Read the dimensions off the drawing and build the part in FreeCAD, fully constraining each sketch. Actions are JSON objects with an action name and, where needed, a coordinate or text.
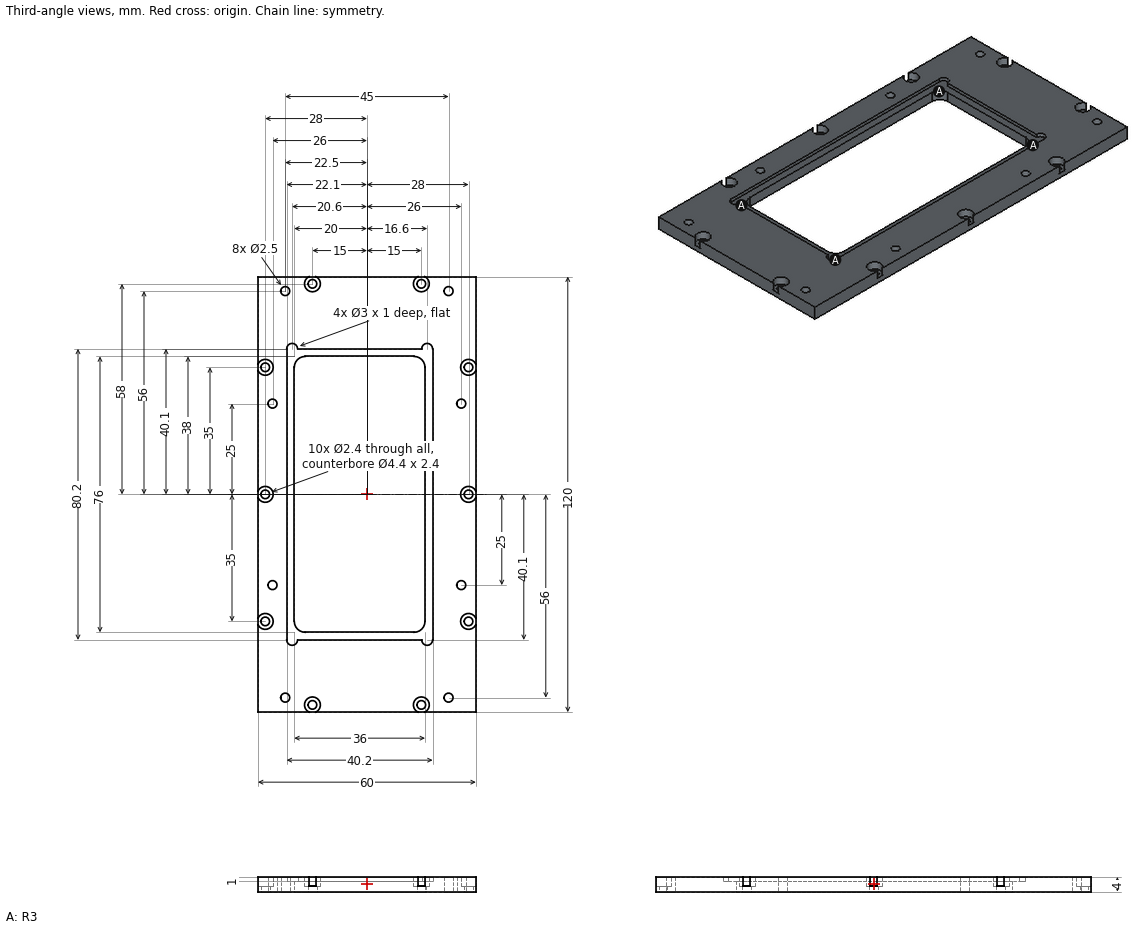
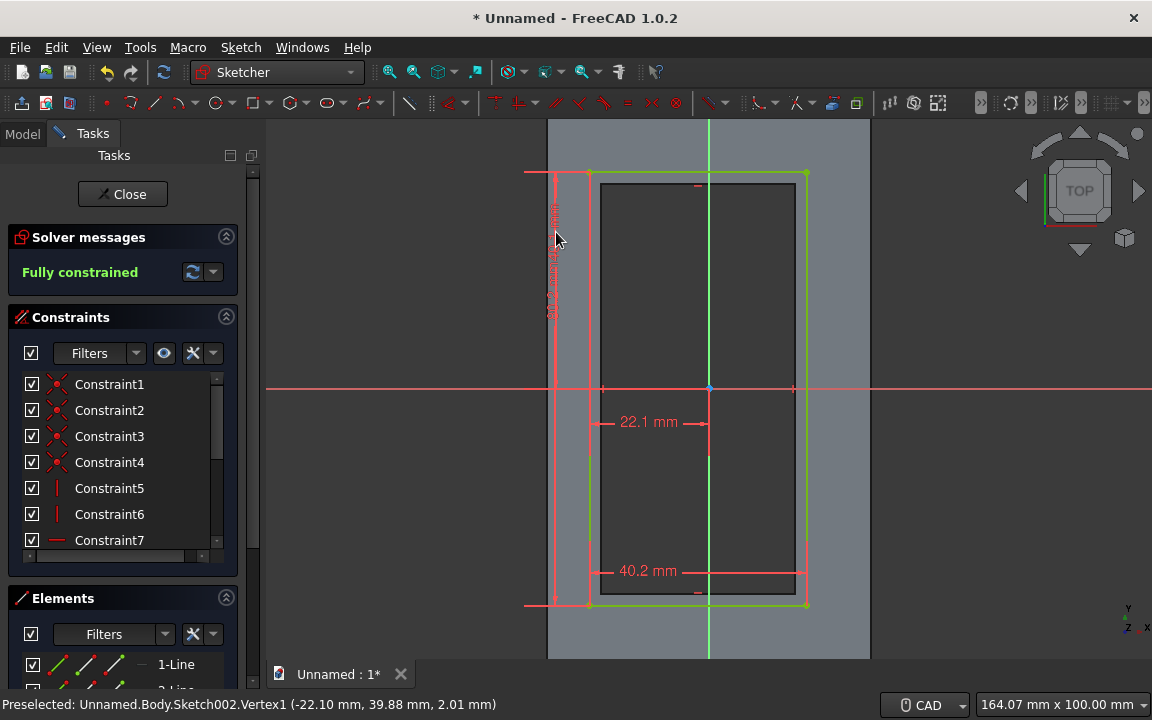
{"action": "left_click", "coordinate": [123, 194]}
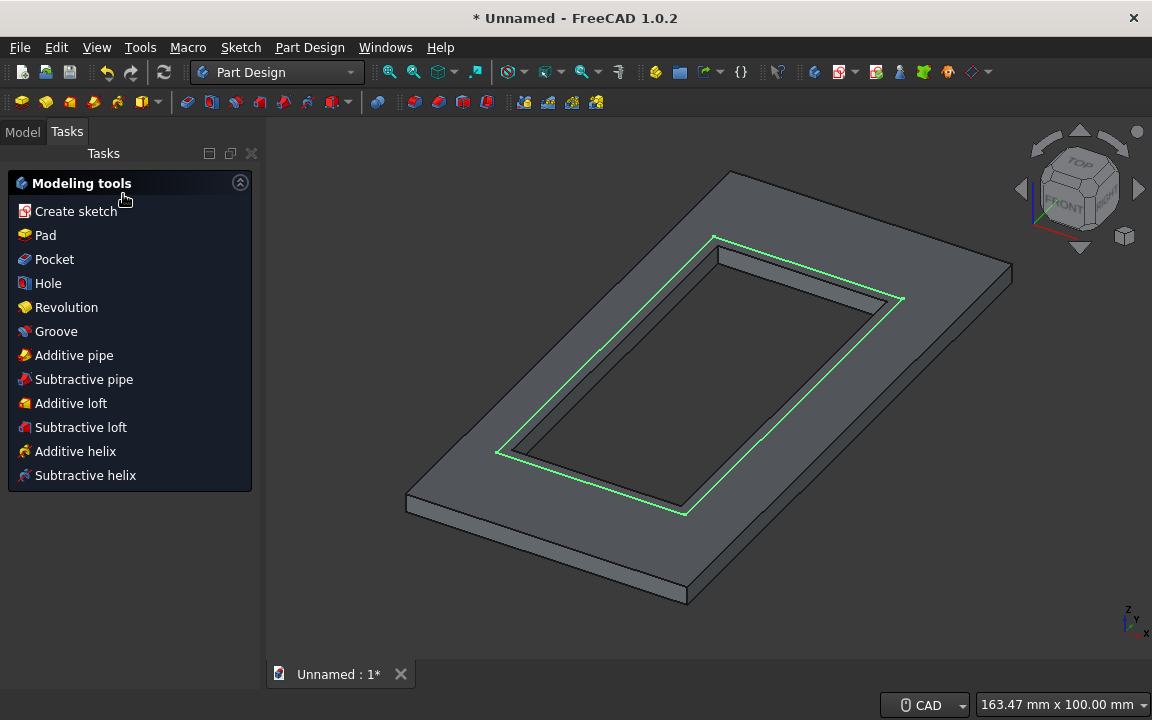
{"action": "left_click", "coordinate": [188, 102]}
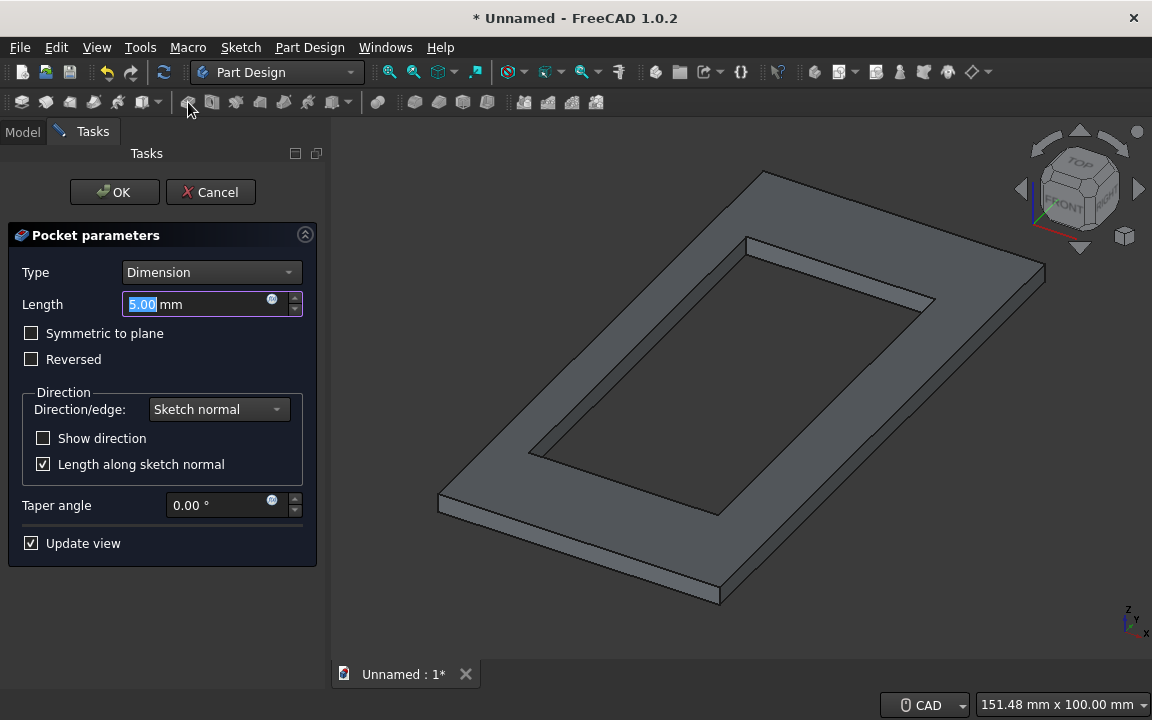
{"action": "type", "text": "1"}
{"action": "key", "text": "Tab"}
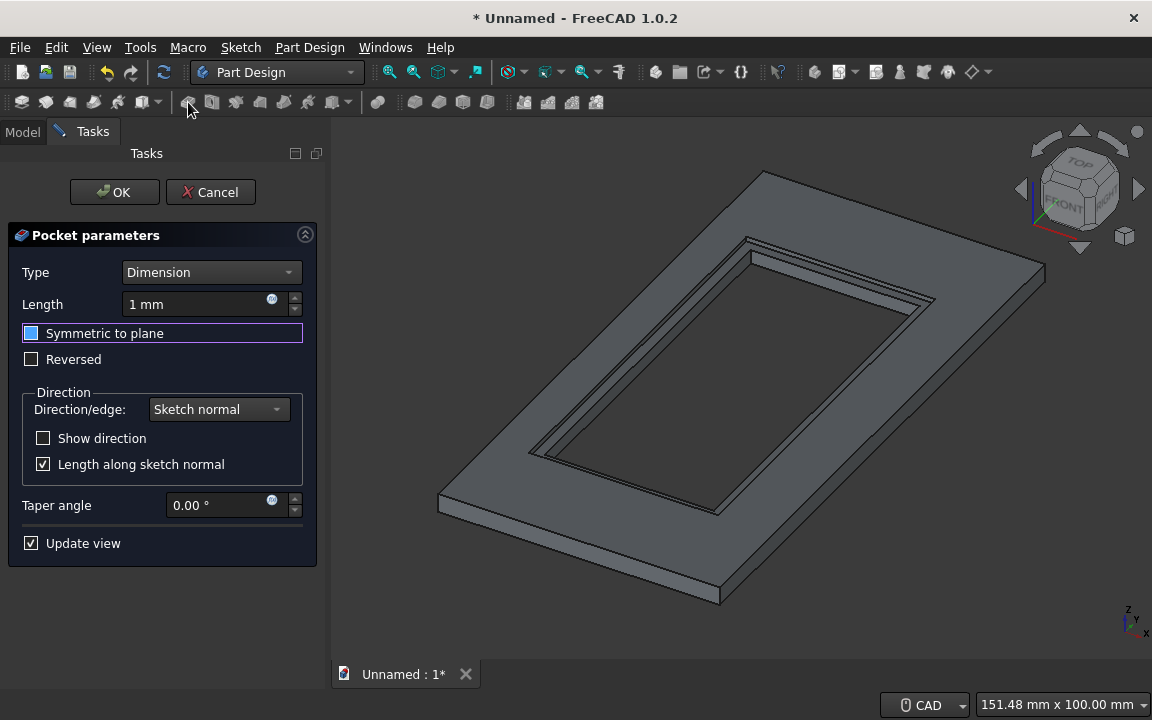
{"action": "left_click", "coordinate": [115, 192]}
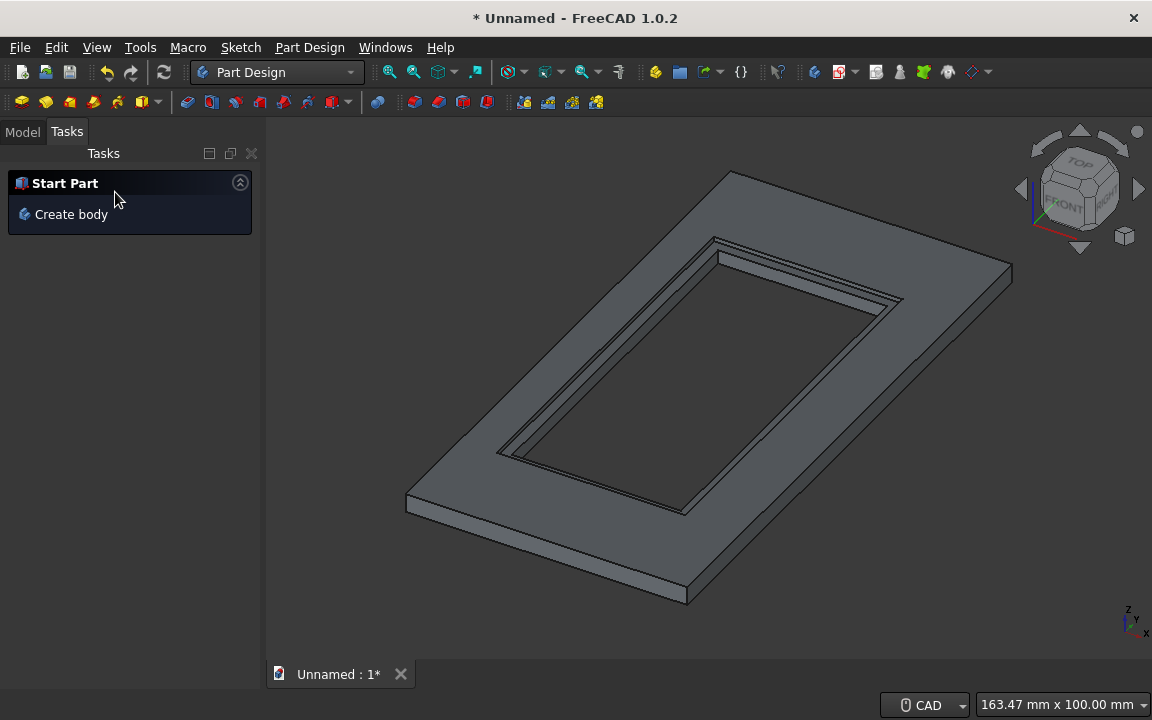
{"action": "left_click", "coordinate": [929, 266]}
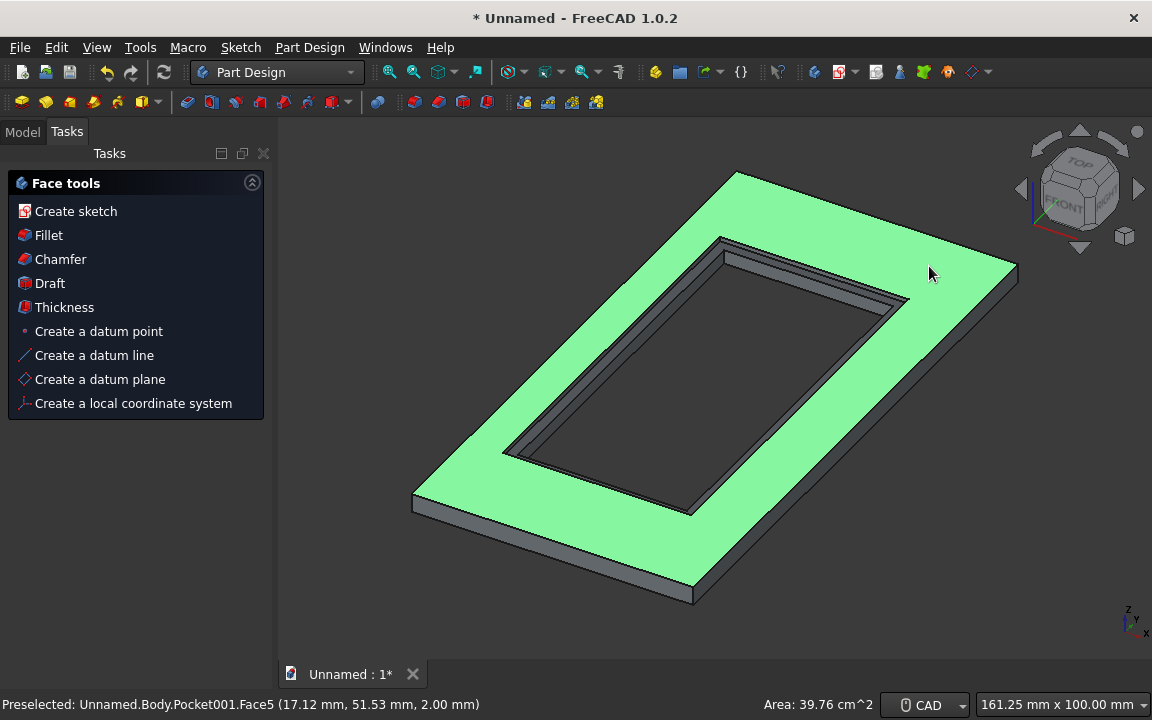
{"action": "left_click", "coordinate": [840, 72]}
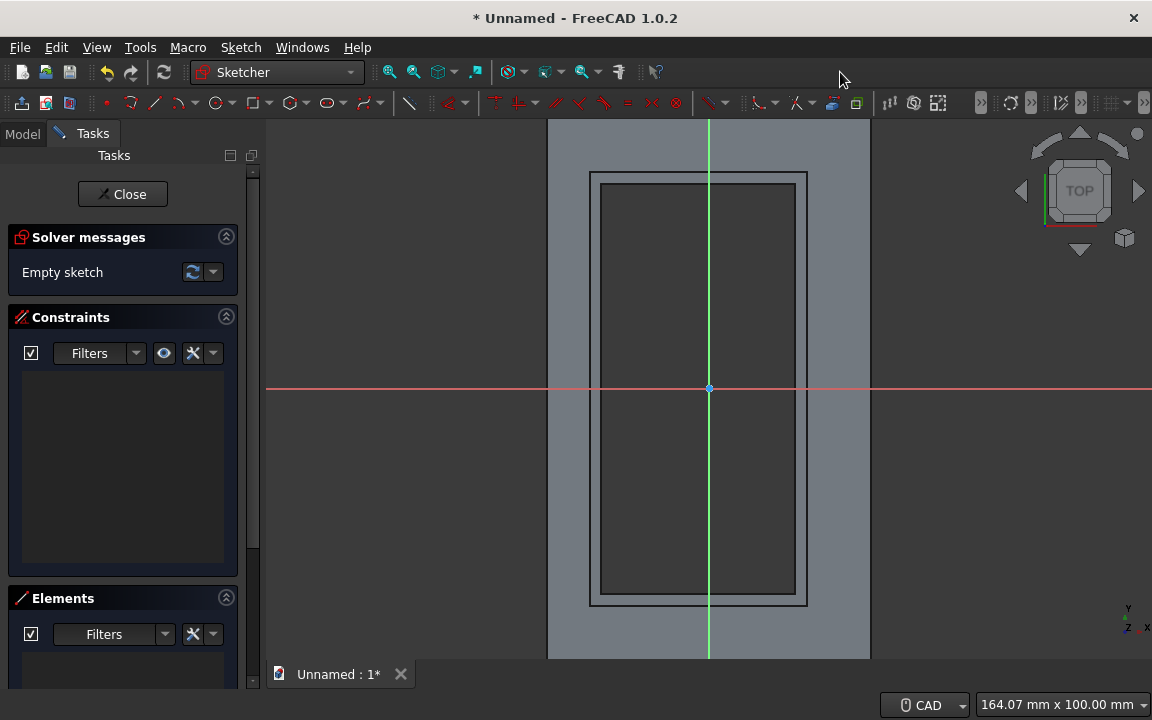
{"action": "scroll", "coordinate": [380, 389], "scroll_direction": "down", "scroll_amount": 1}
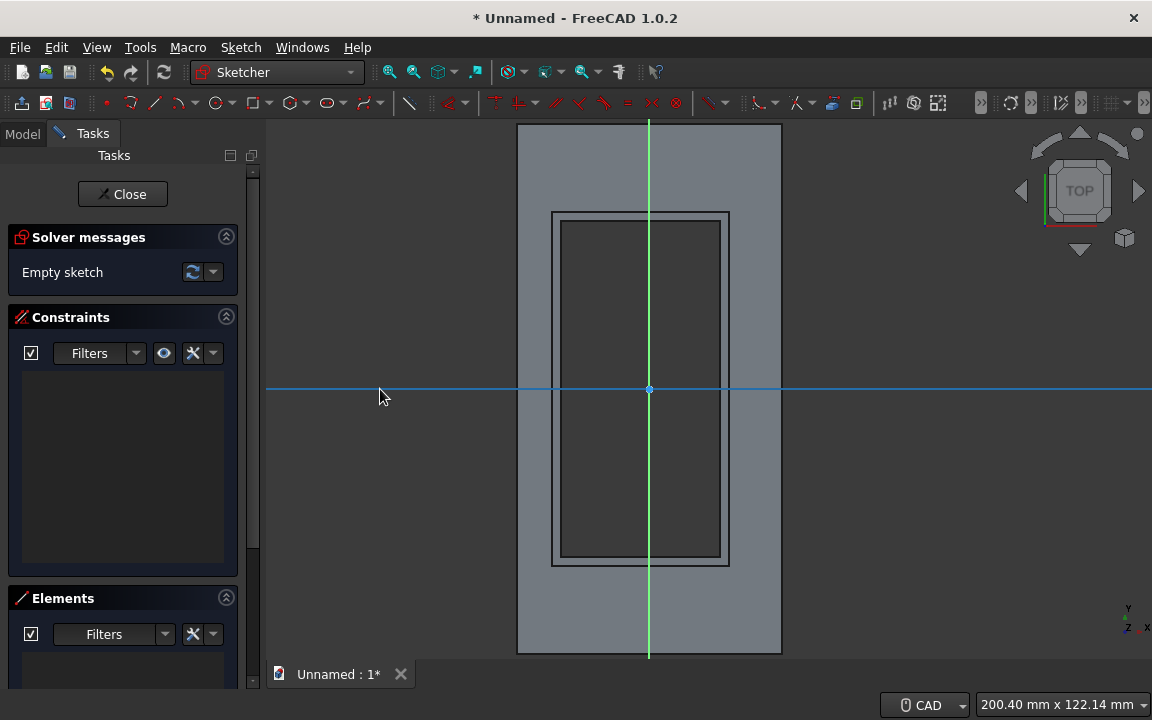
{"action": "key", "text": "g c"}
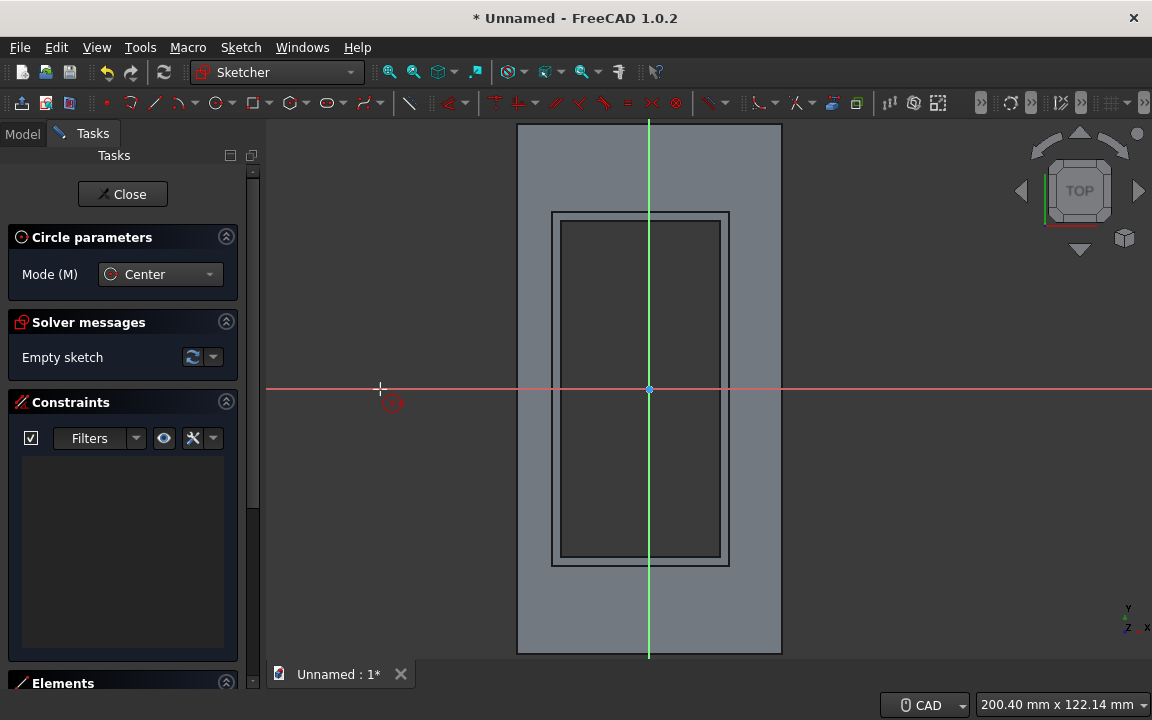
{"action": "scroll", "coordinate": [558, 212], "scroll_direction": "up", "scroll_amount": 7}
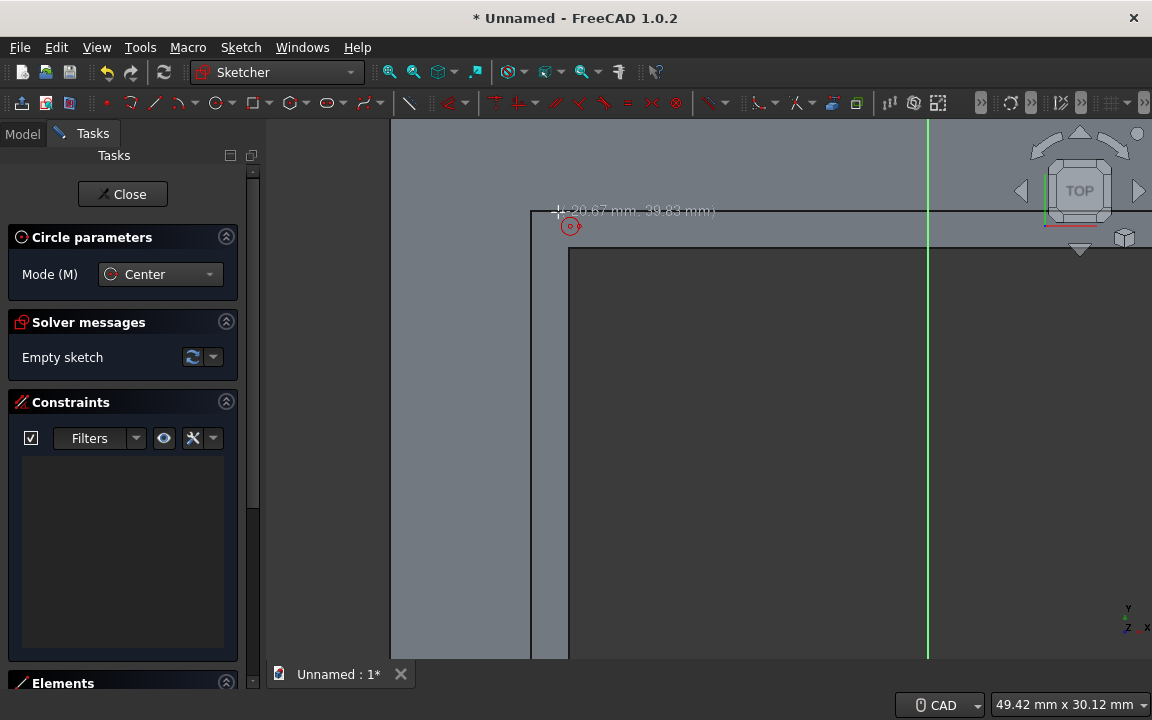
{"action": "scroll", "coordinate": [558, 212], "scroll_direction": "down", "scroll_amount": 7}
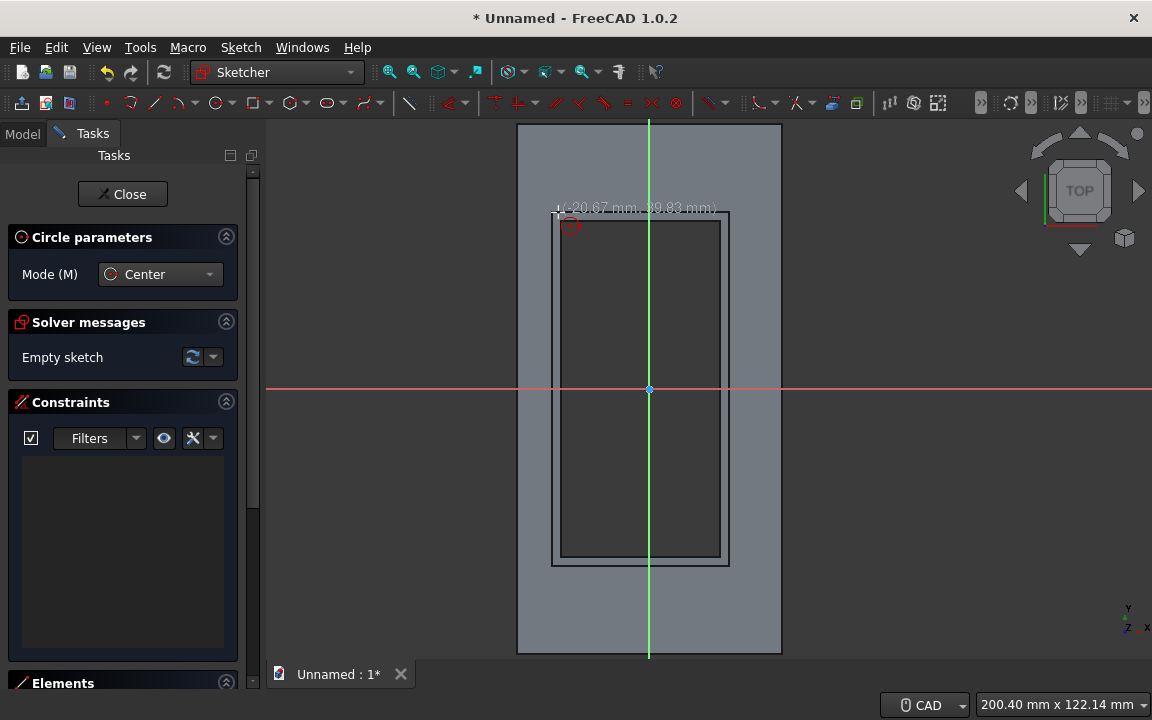
{"action": "left_click", "coordinate": [558, 212]}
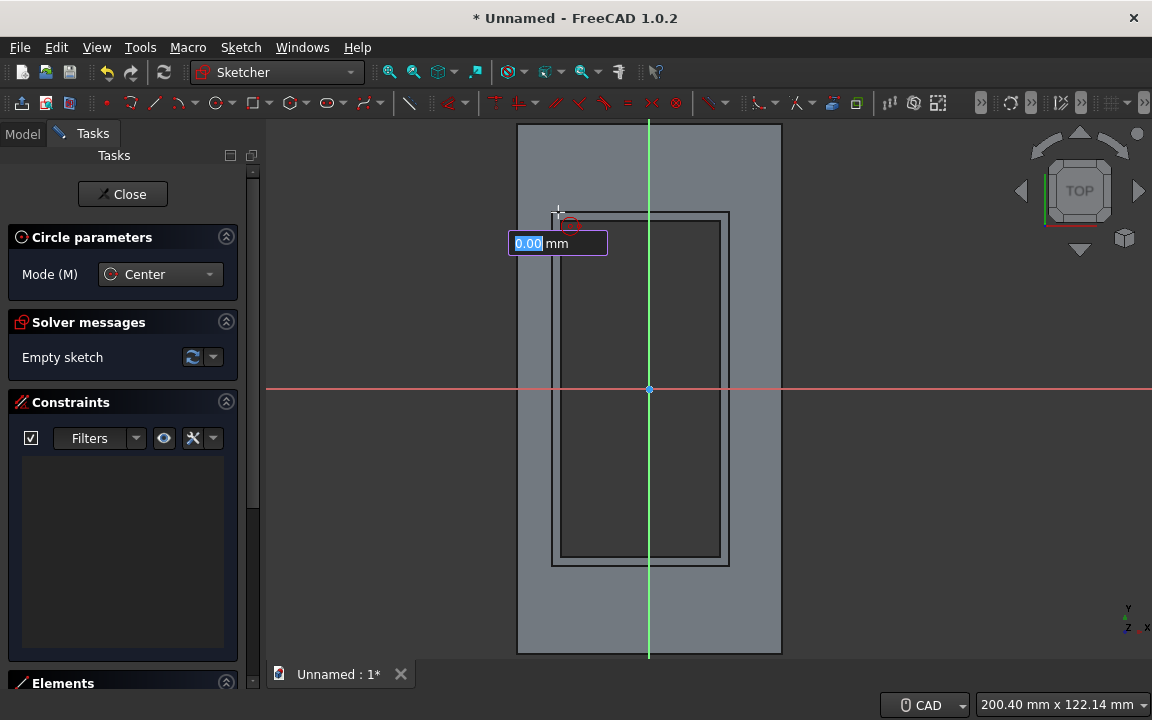
{"action": "scroll", "coordinate": [563, 207], "scroll_direction": "up", "scroll_amount": 5}